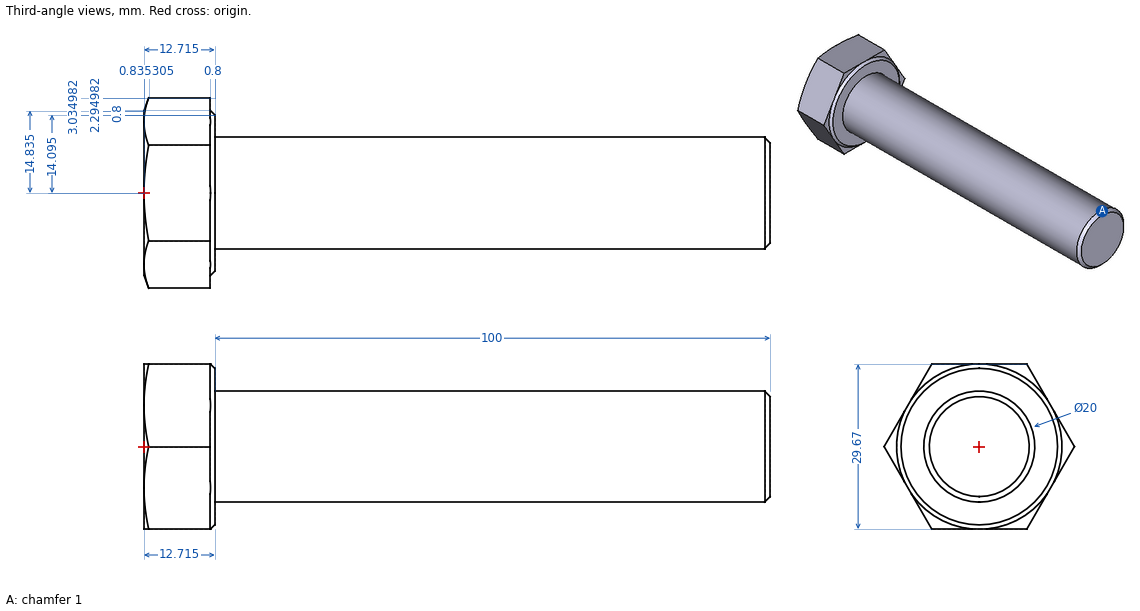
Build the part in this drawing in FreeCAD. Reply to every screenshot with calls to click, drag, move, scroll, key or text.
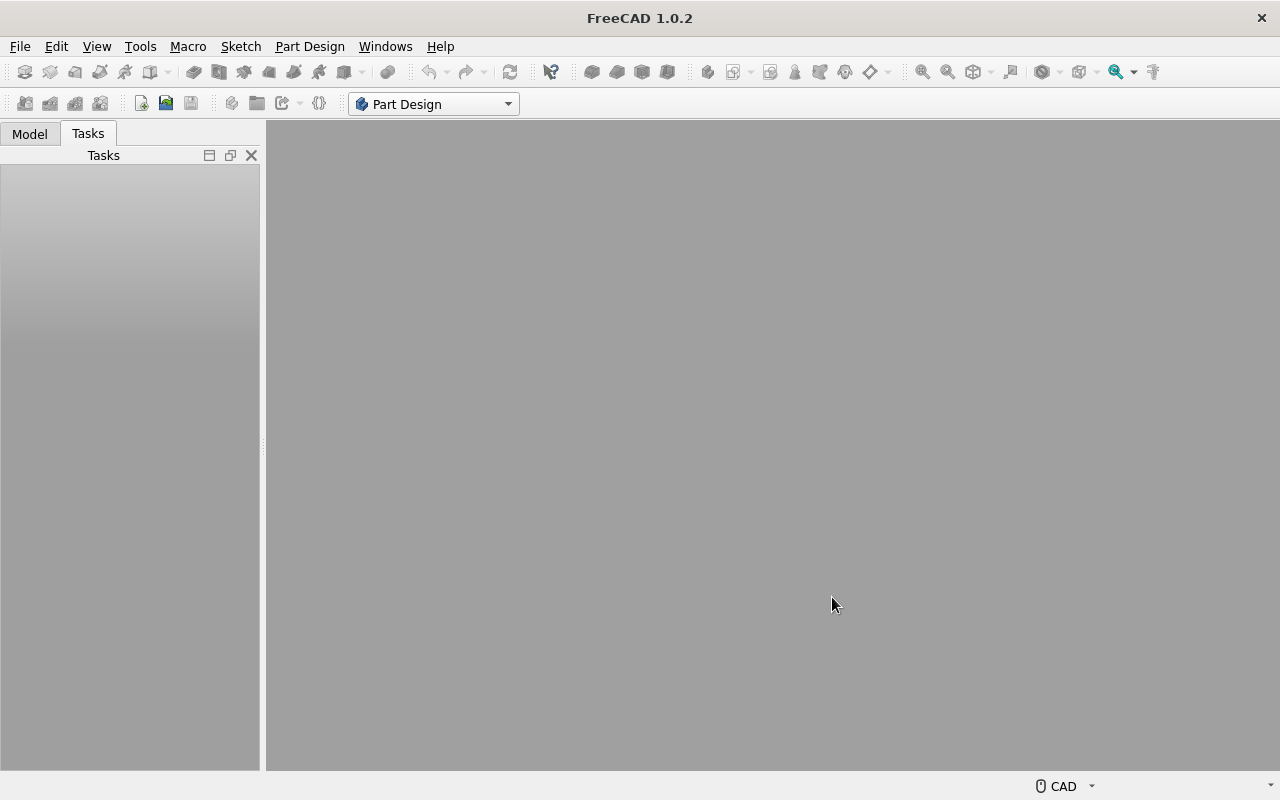
key(ctrl+n)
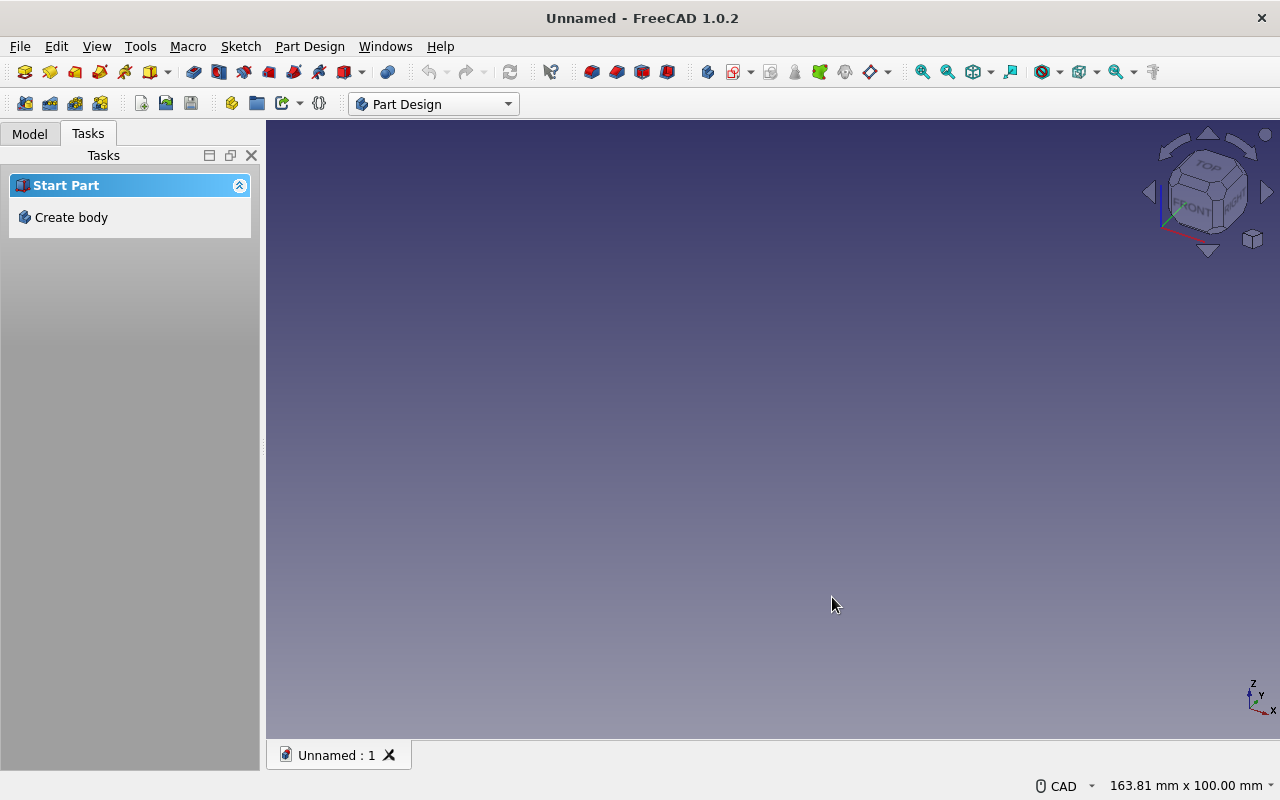
click(732, 72)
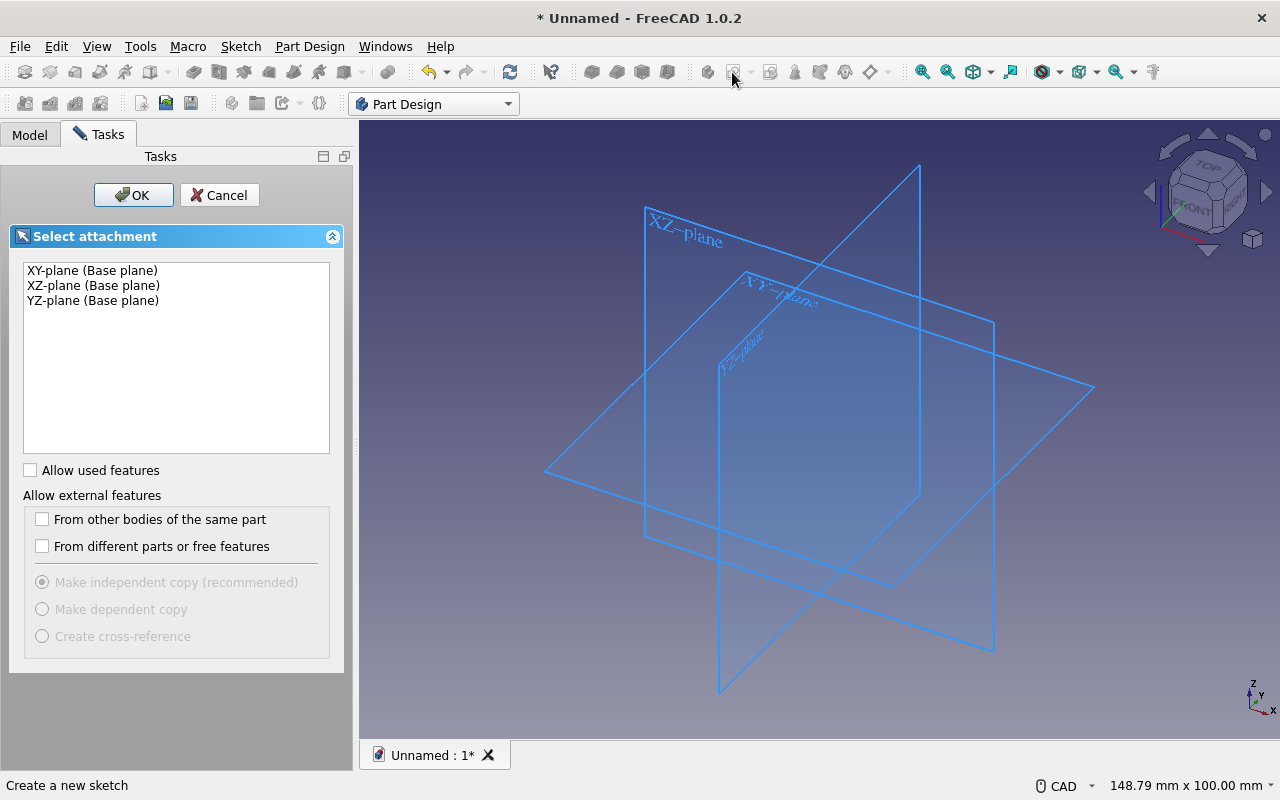
click(84, 300)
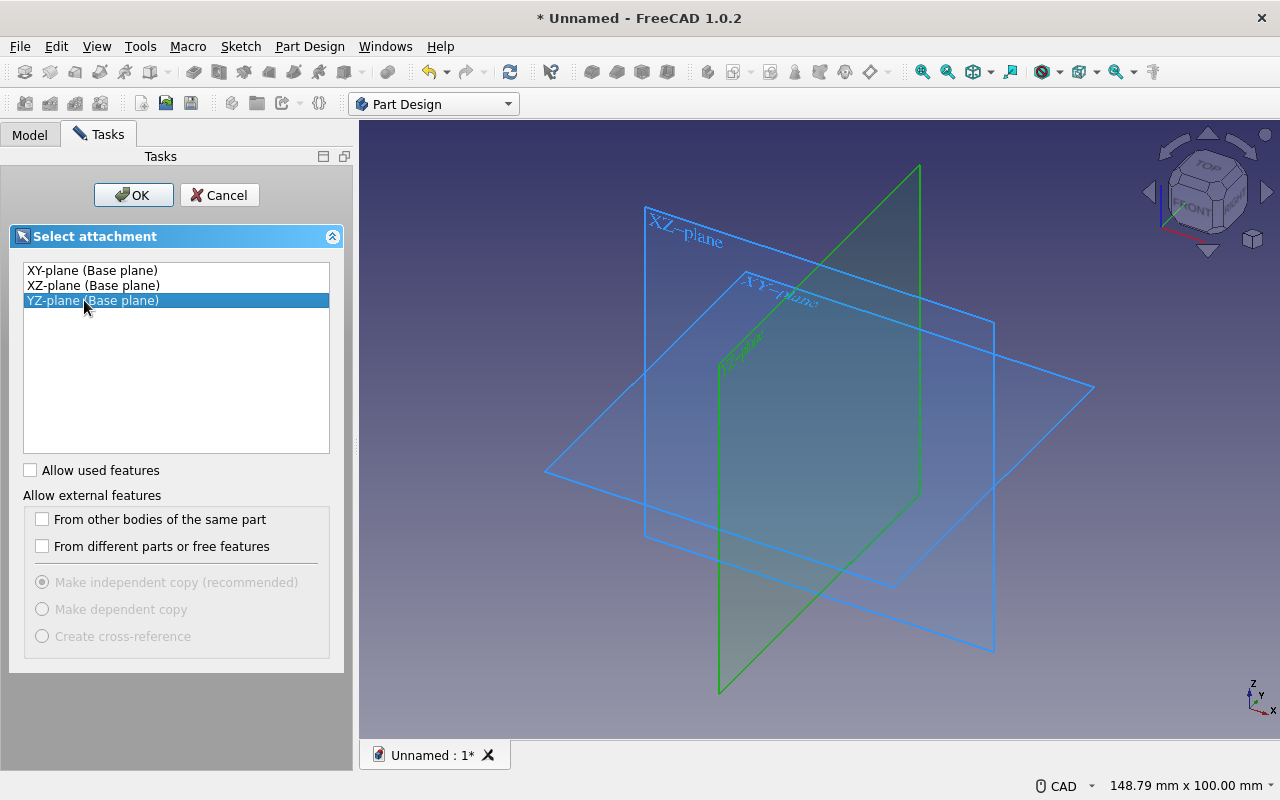
click(134, 195)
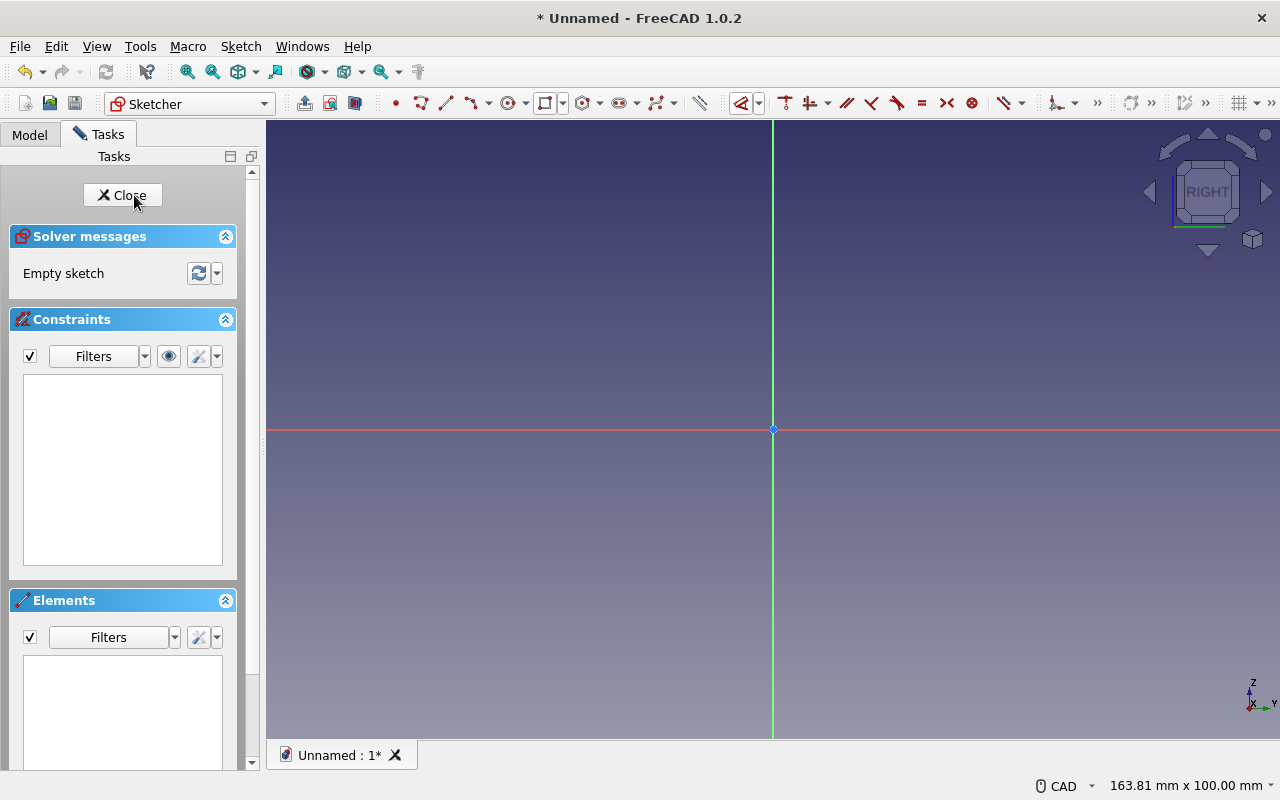
scroll(829, 430, up, 4)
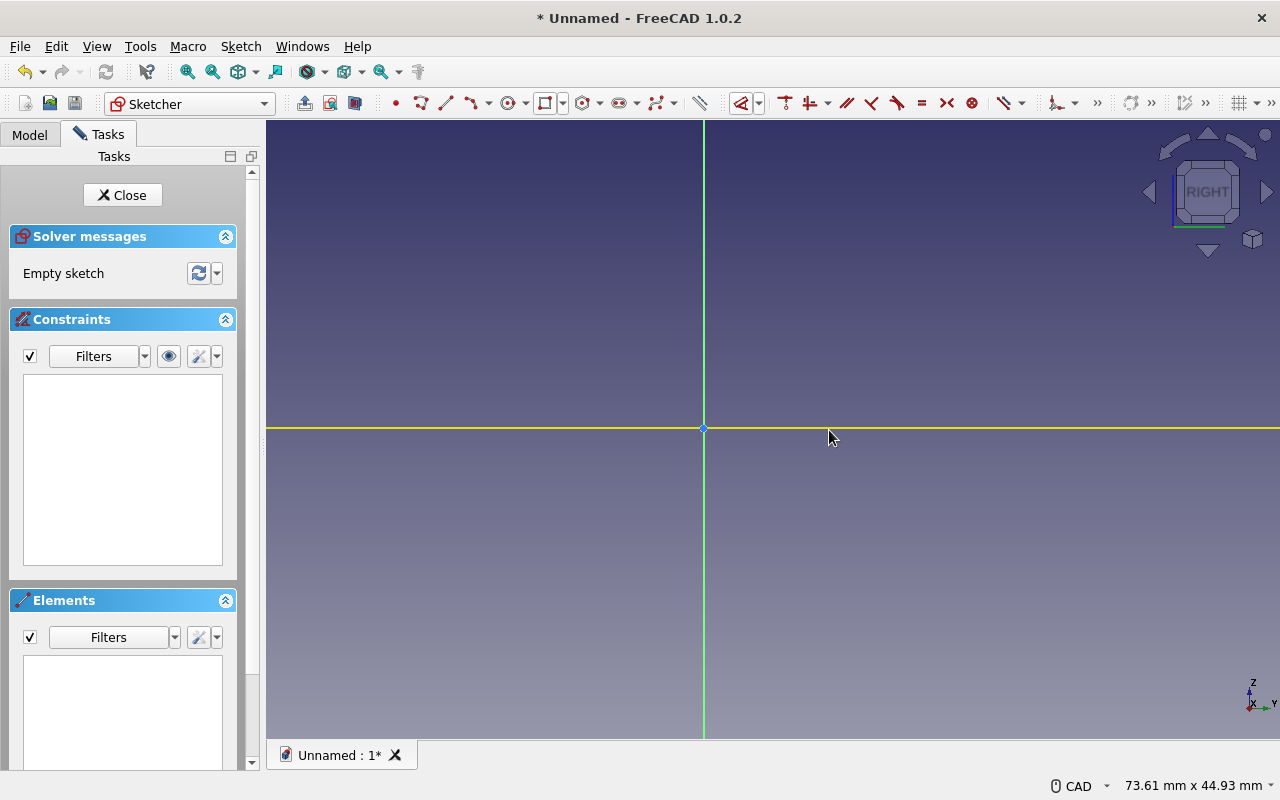
key(g)
key(p)
key(6)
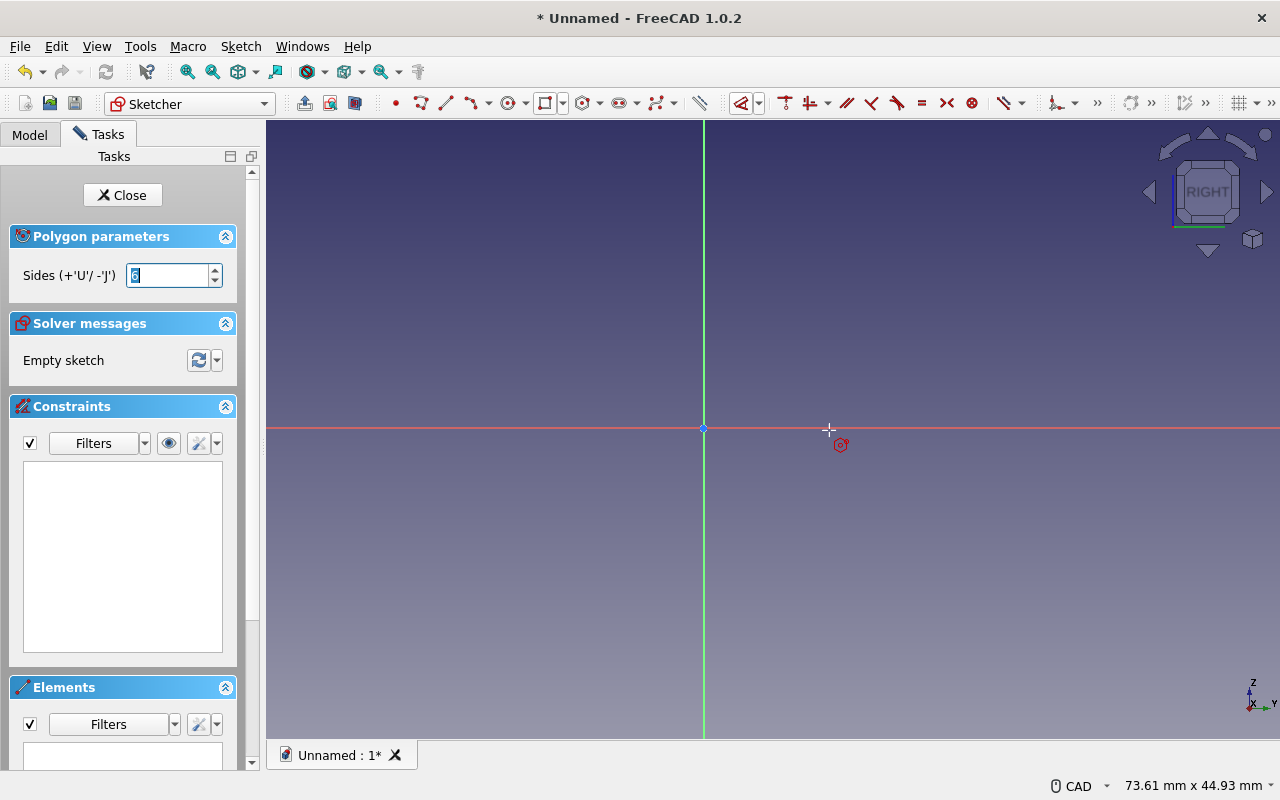
click(704, 428)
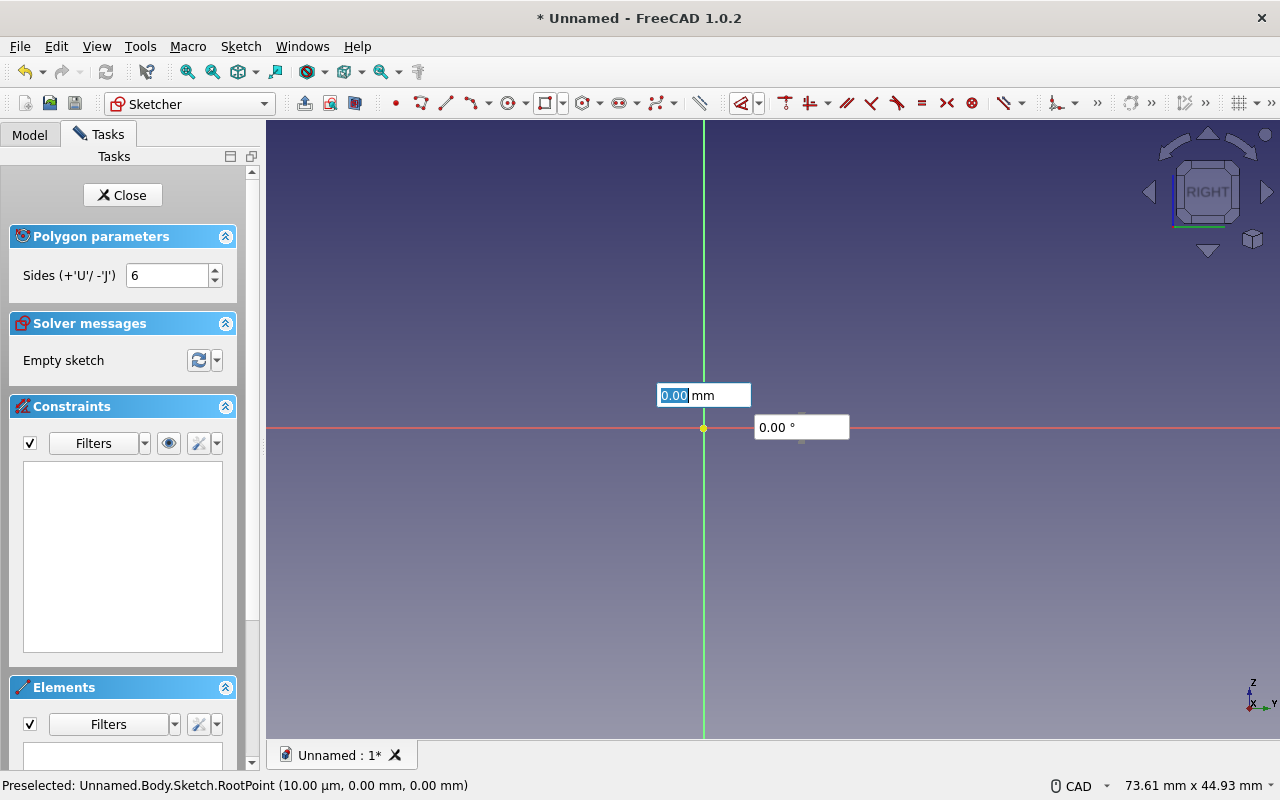
click(940, 428)
key(Escape)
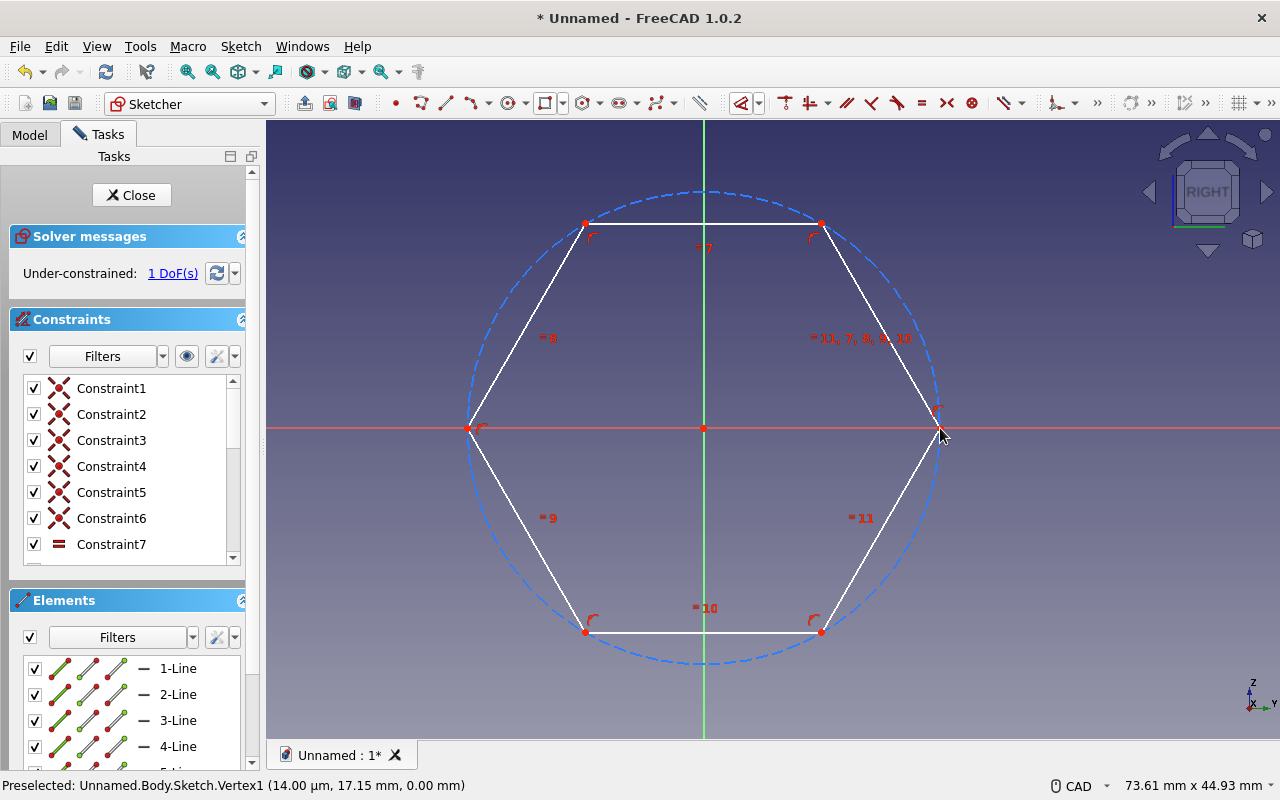
key(d)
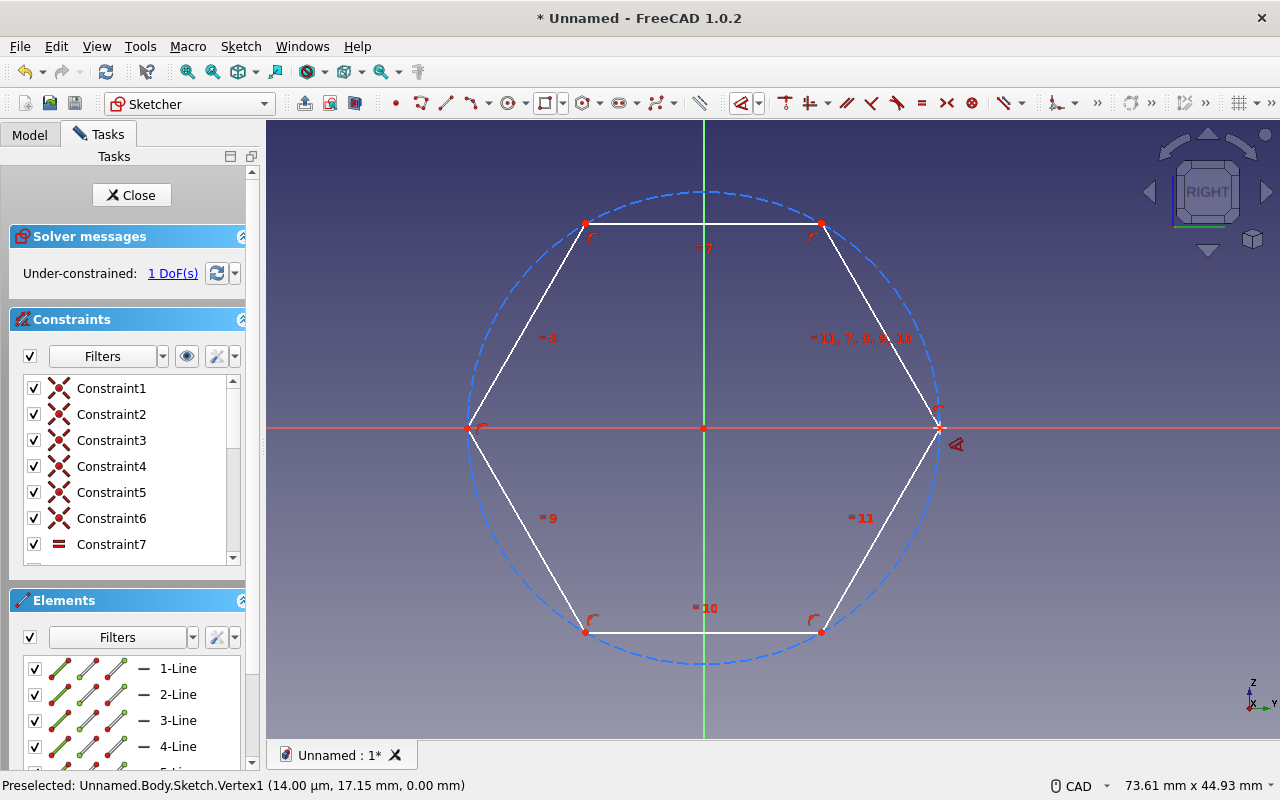
click(586, 633)